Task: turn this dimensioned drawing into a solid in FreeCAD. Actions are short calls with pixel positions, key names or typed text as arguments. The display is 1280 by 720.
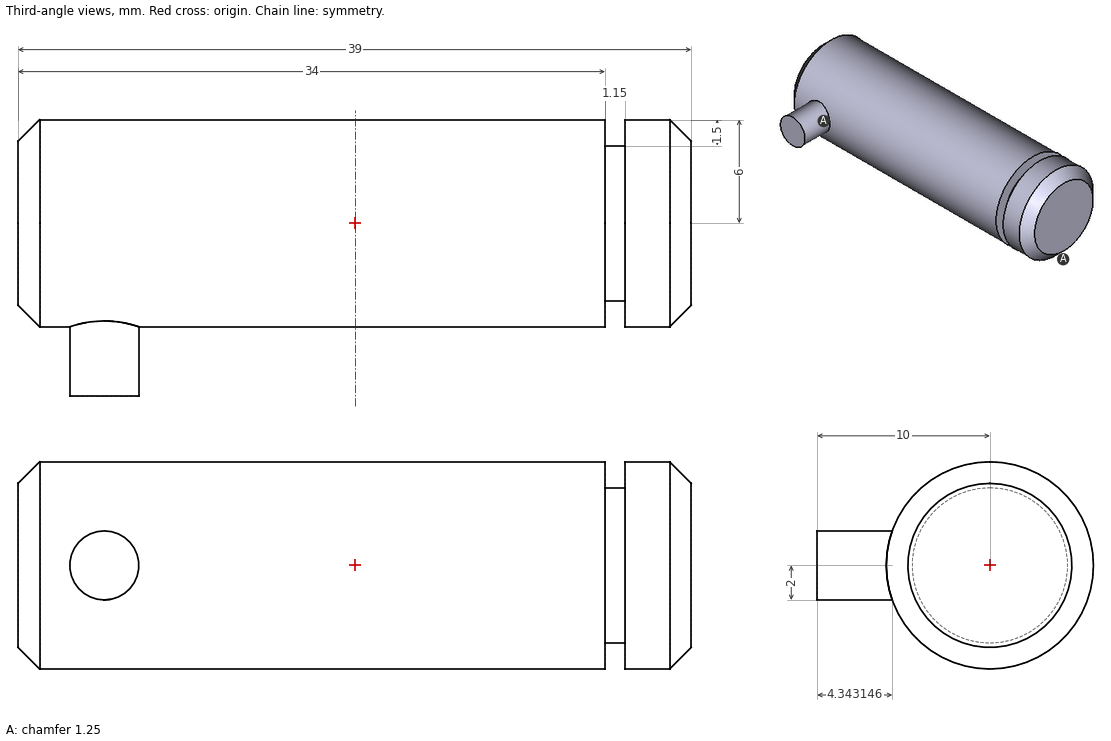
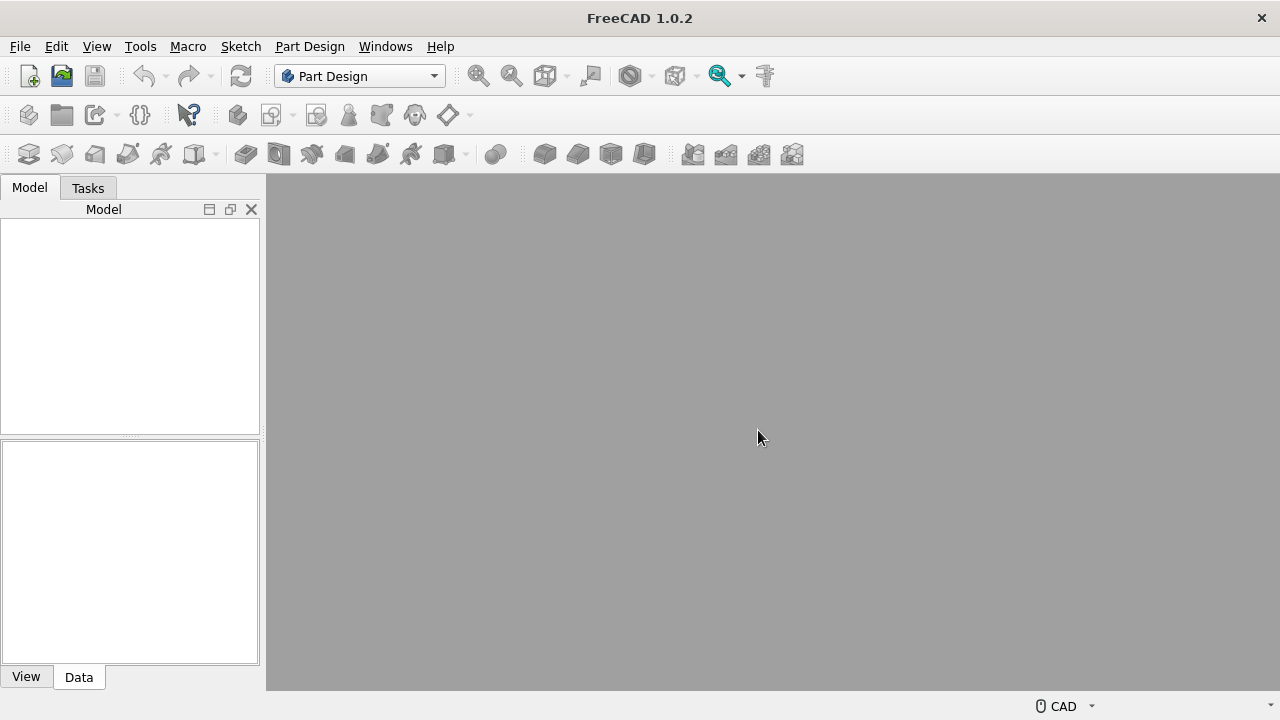
key(ctrl+n)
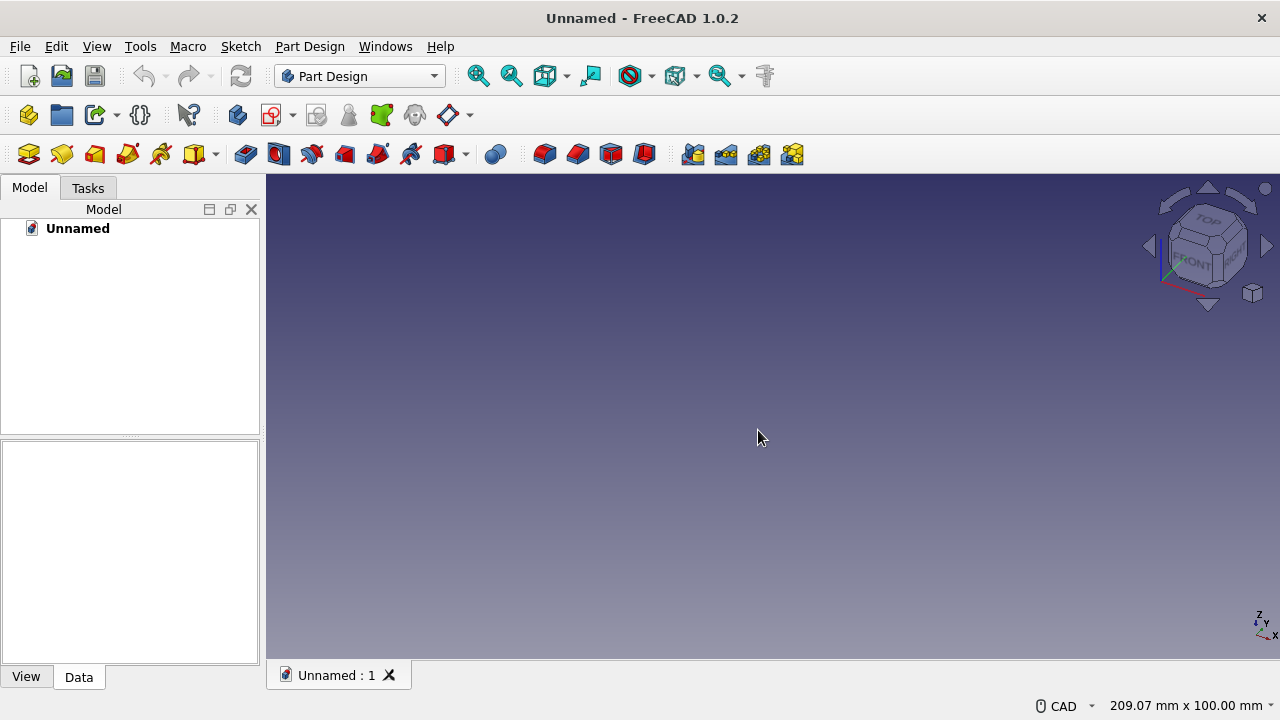
click(270, 116)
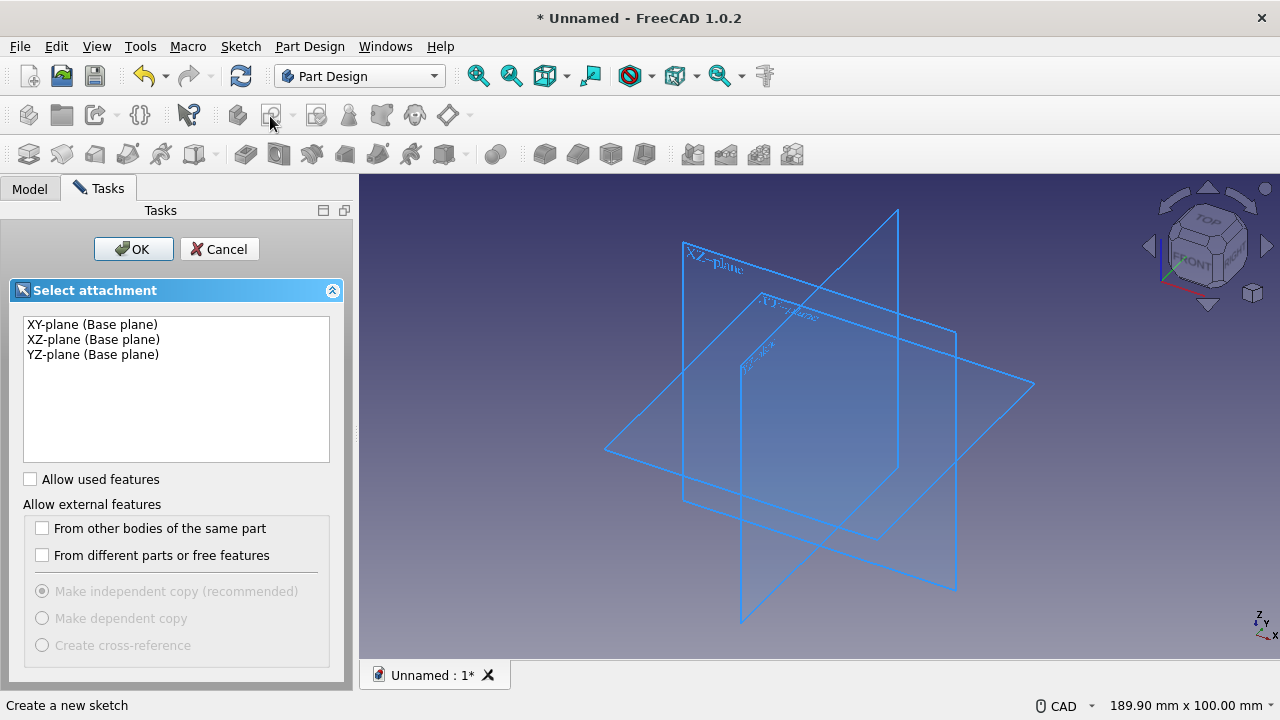
click(84, 324)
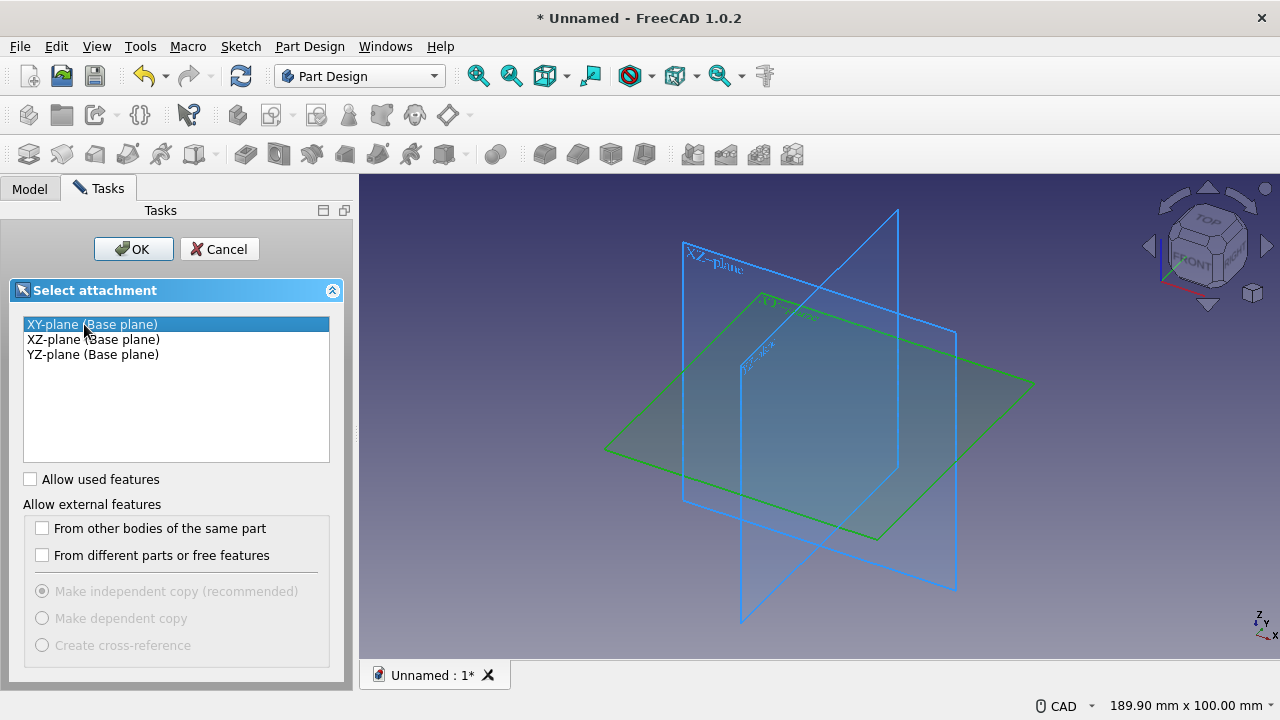
click(134, 249)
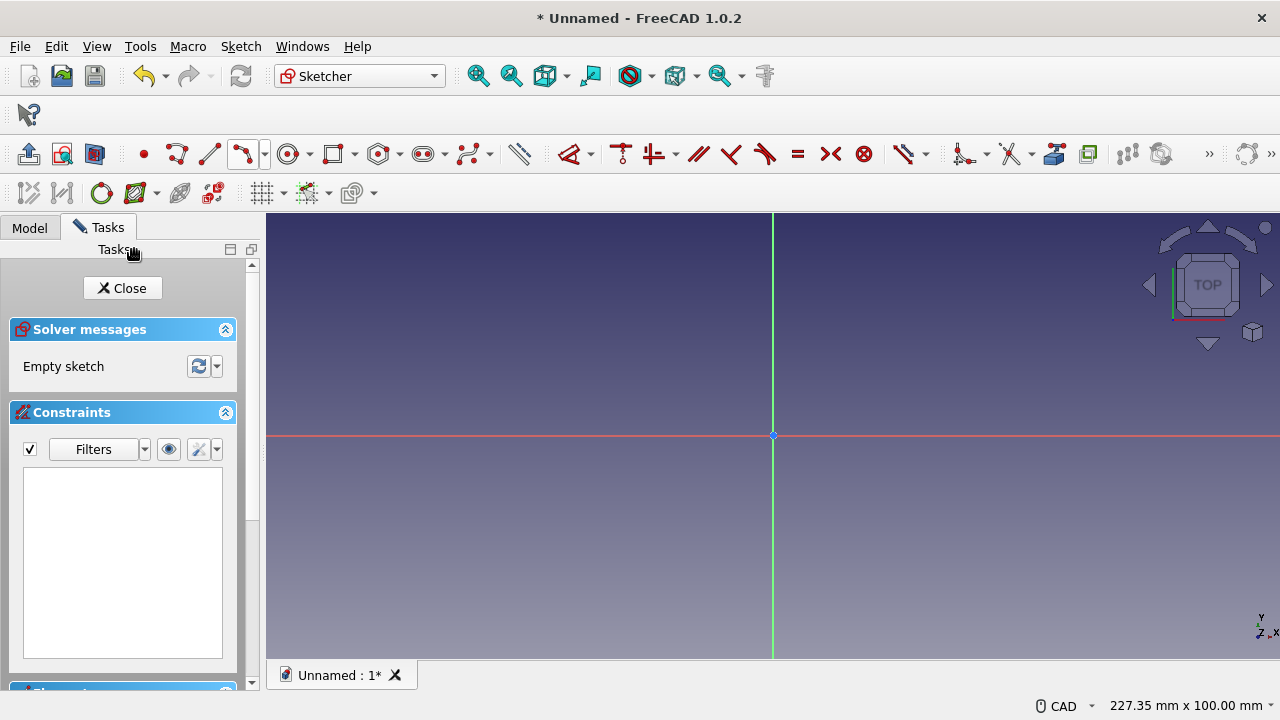
scroll(803, 417, up, 6)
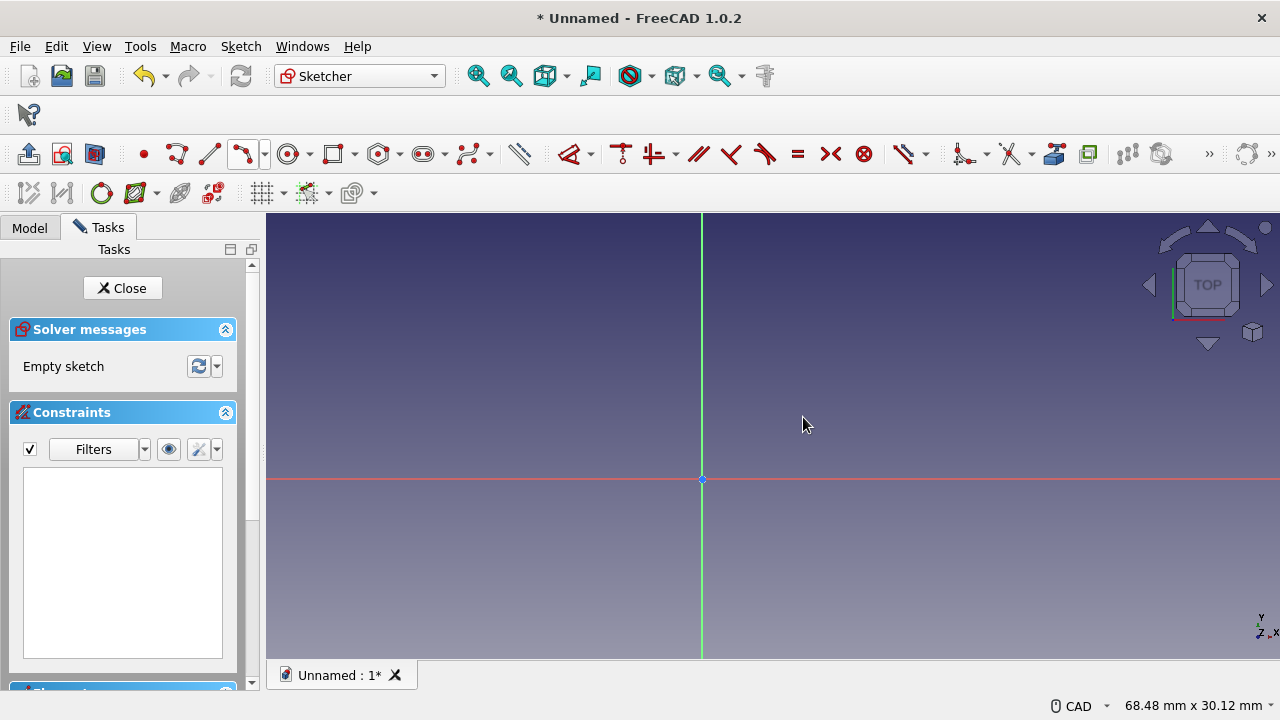
key(g)
key(m)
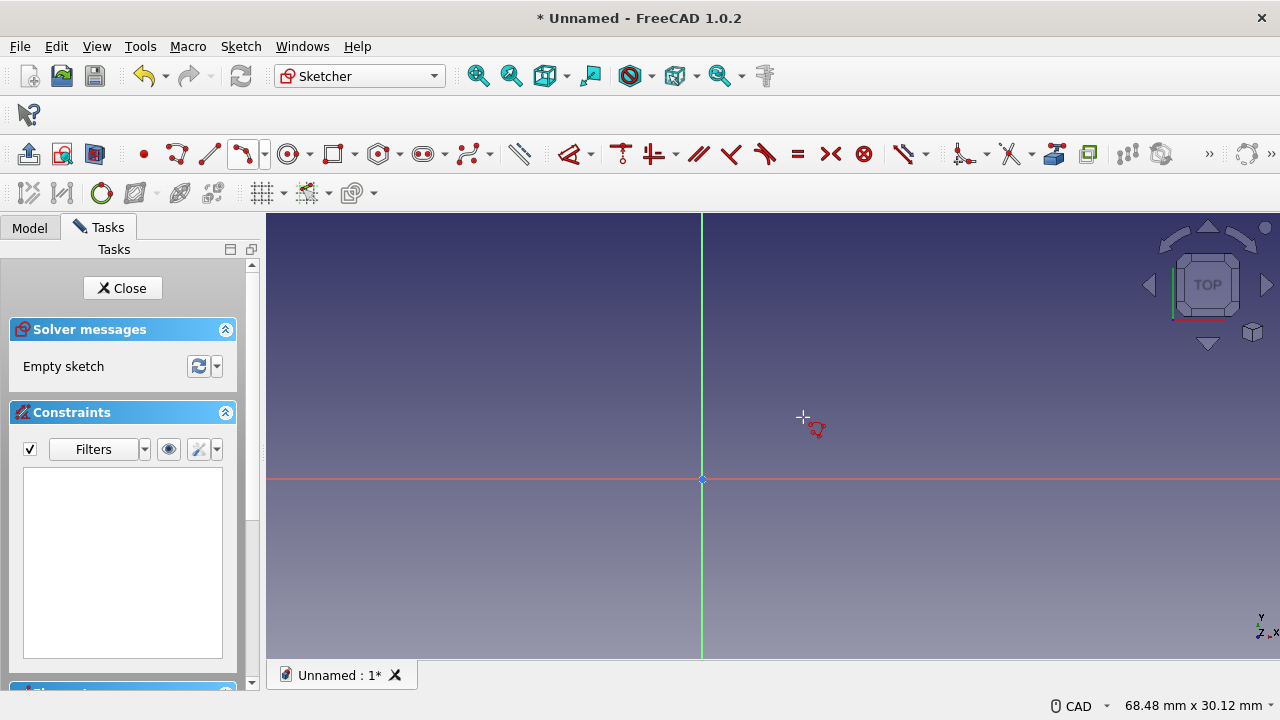
click(917, 412)
click(934, 412)
click(934, 390)
click(991, 390)
click(991, 479)
click(413, 470)
click(413, 390)
click(917, 390)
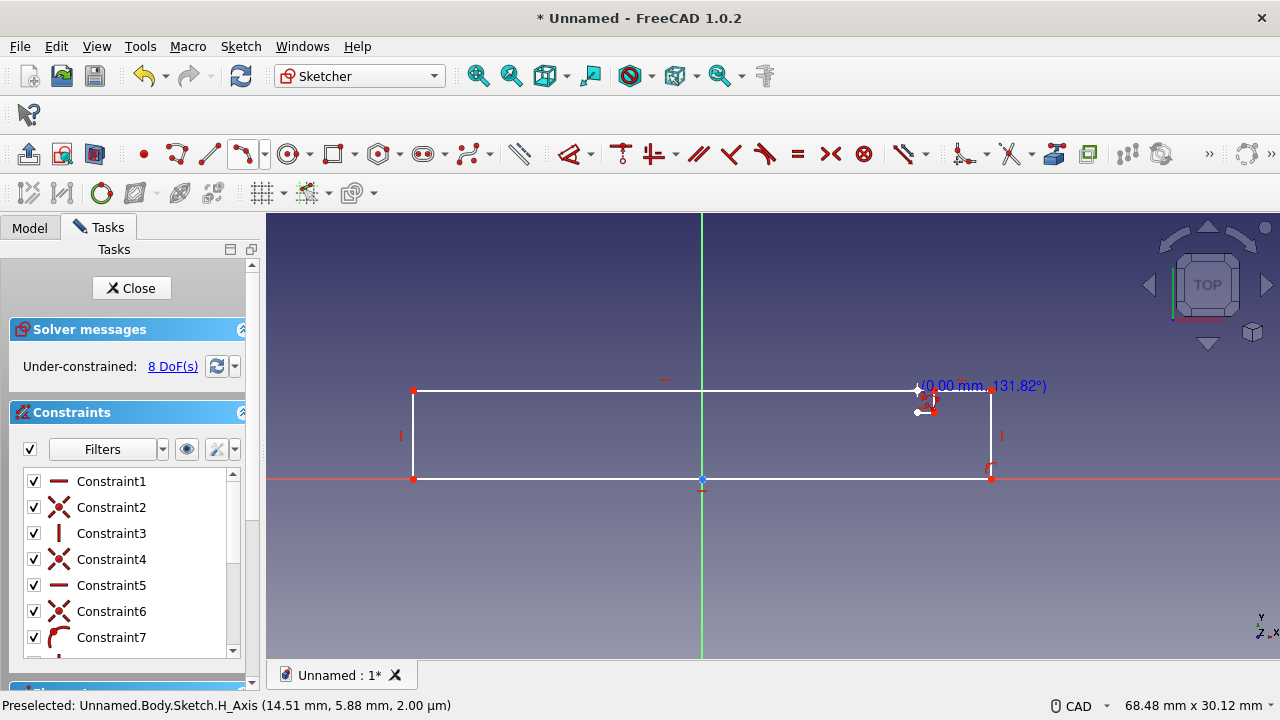
scroll(917, 412, up, 4)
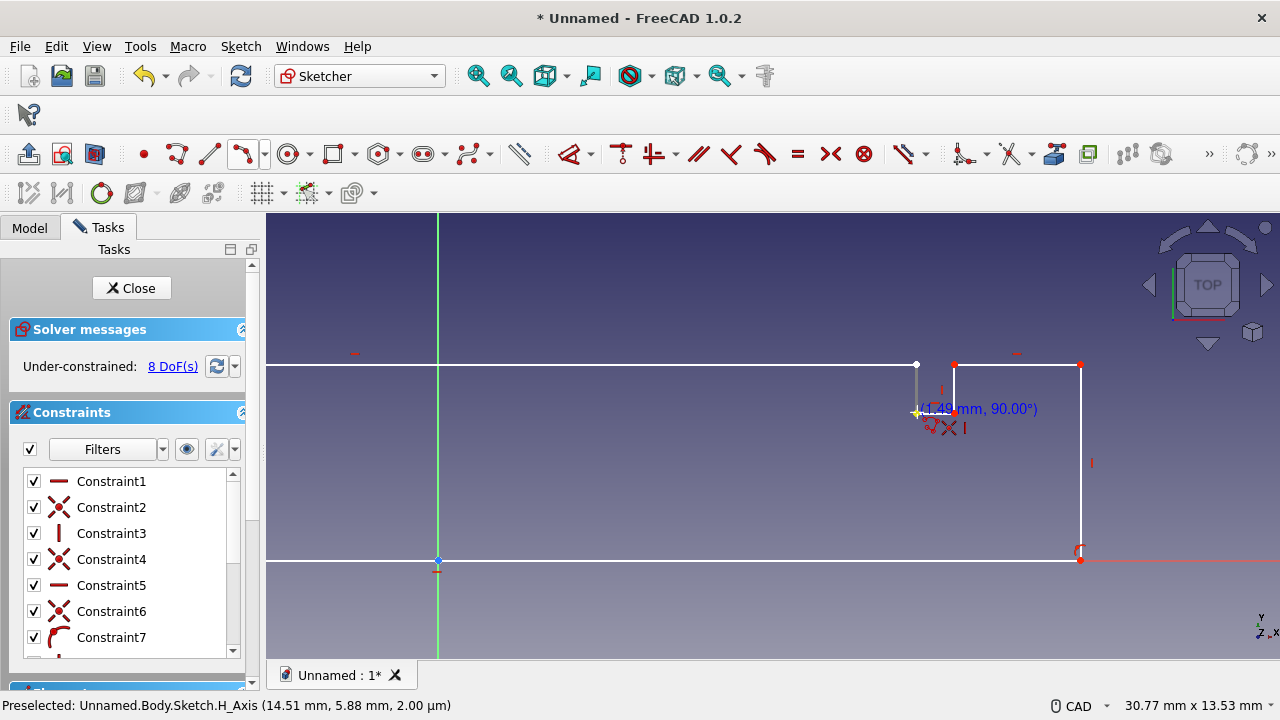
click(916, 414)
key(Escape)
key(Escape)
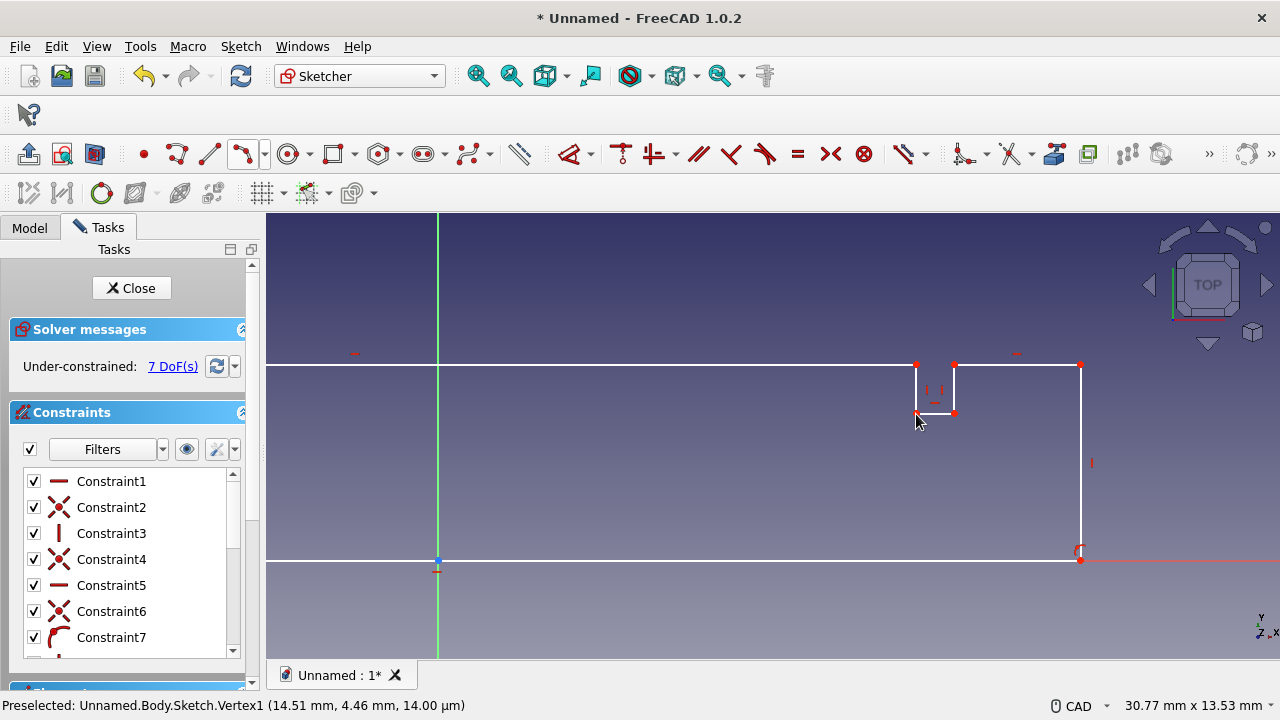
click(1081, 365)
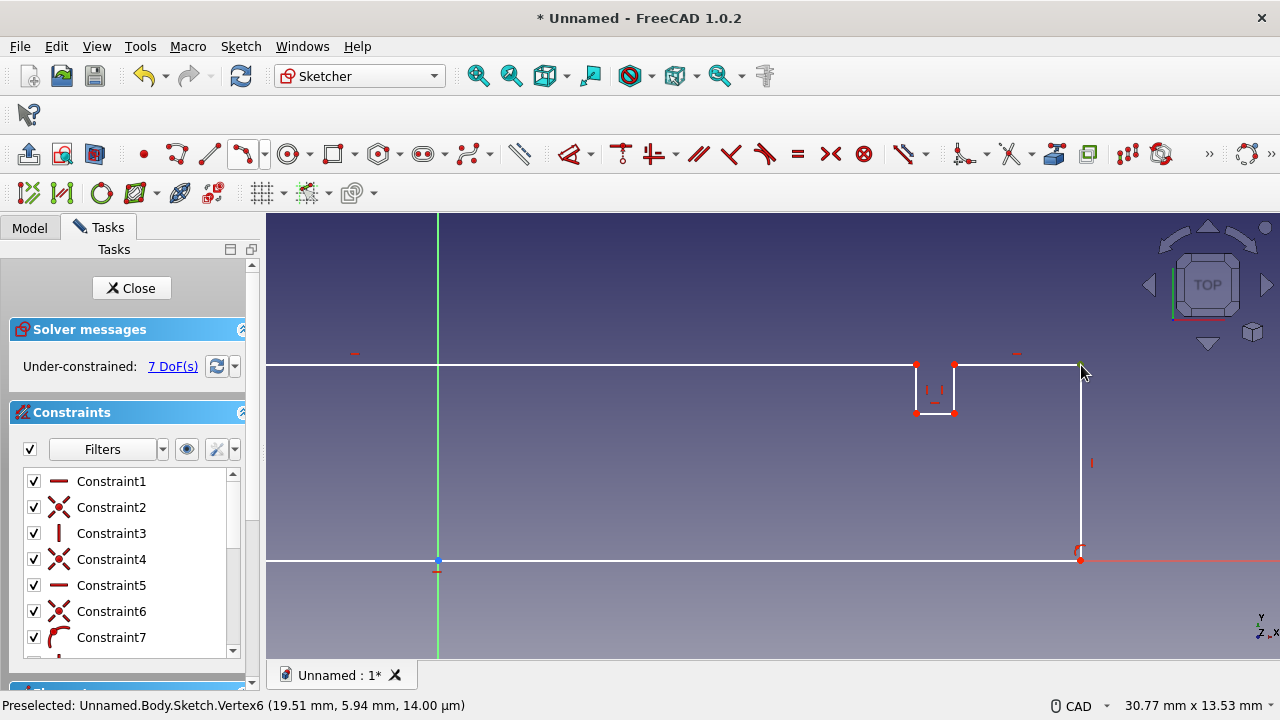
scroll(922, 415, down, 4)